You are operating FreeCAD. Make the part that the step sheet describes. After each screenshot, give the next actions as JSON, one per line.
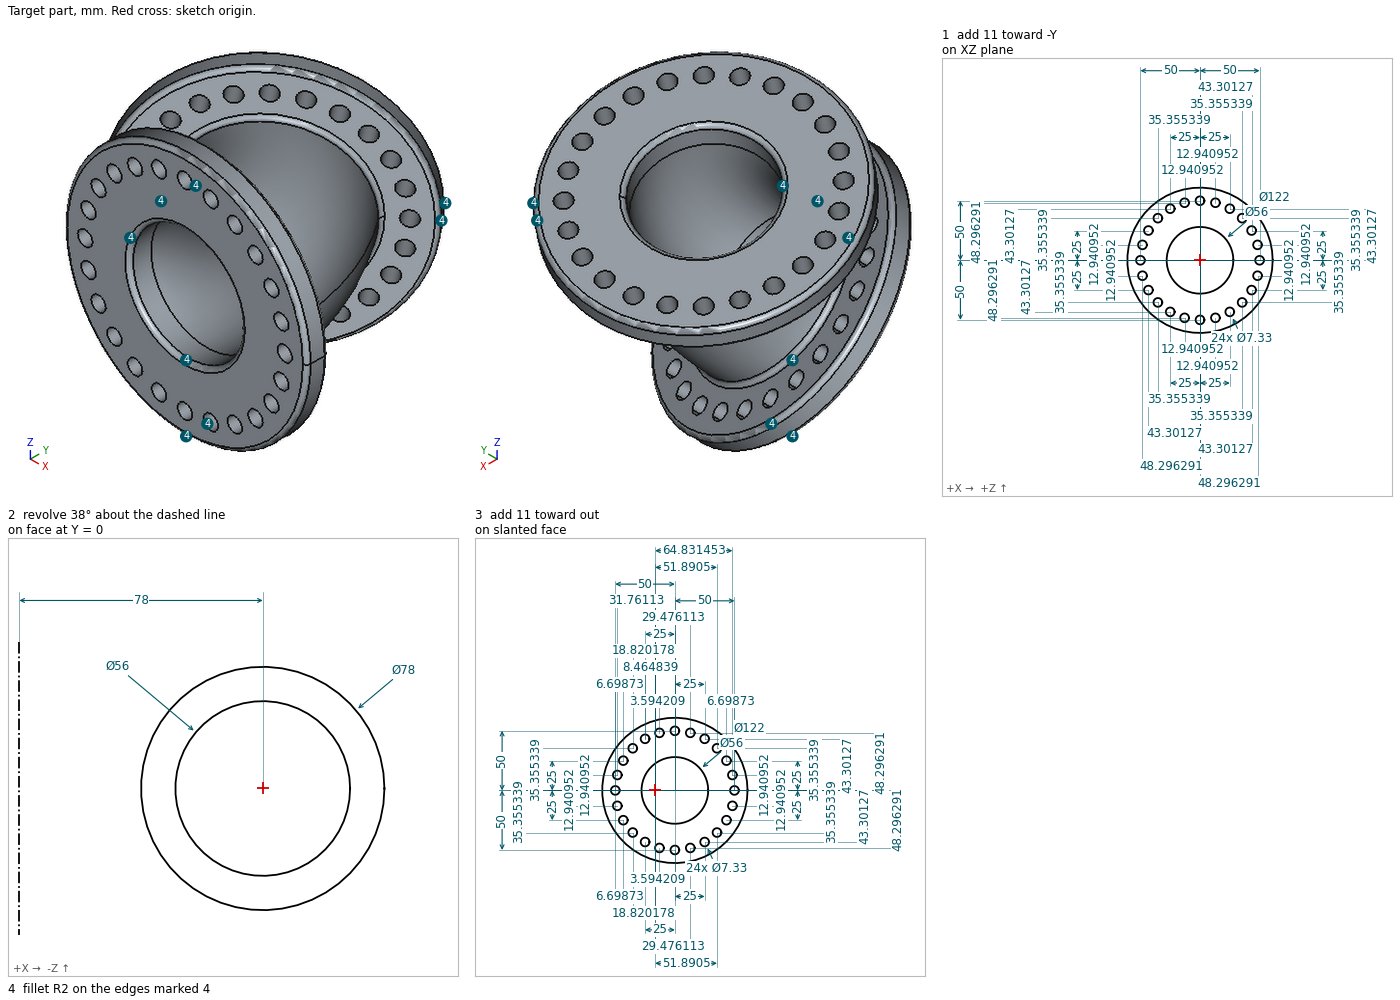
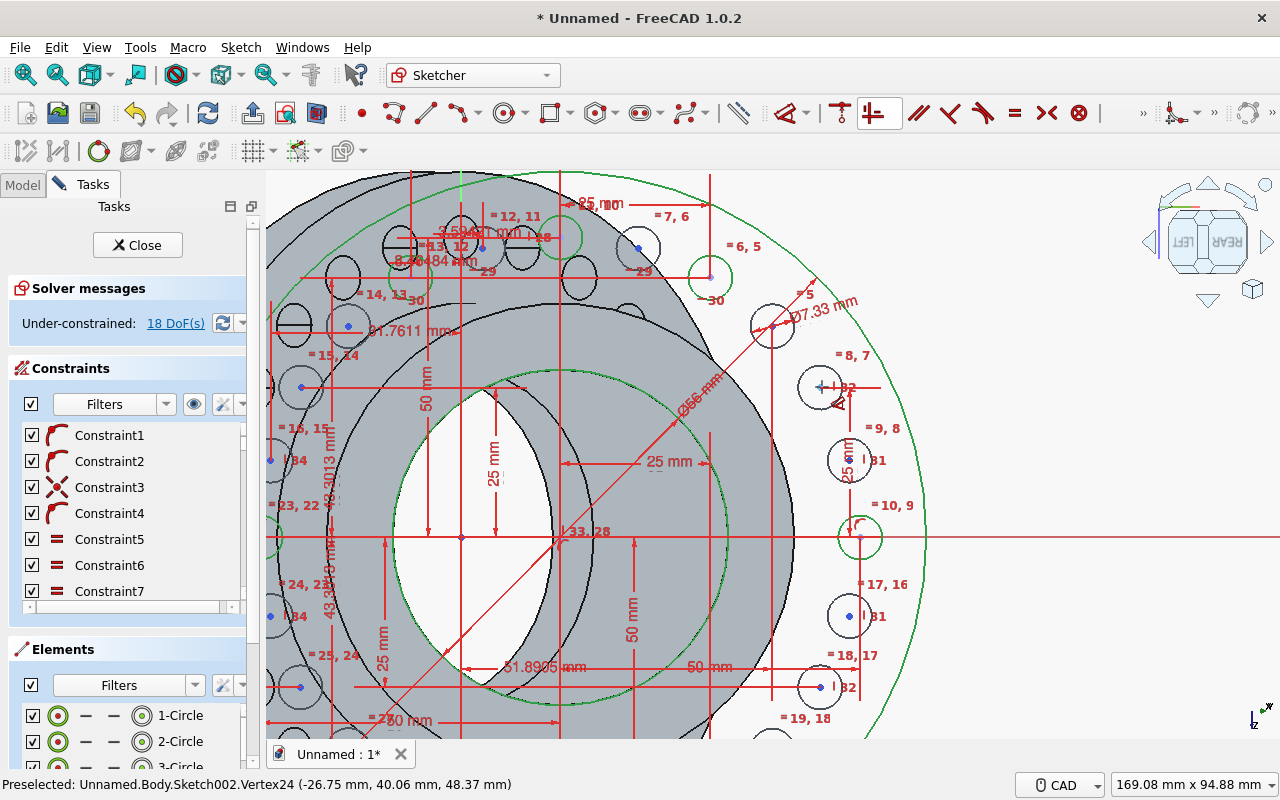
{"action": "left_click", "coordinate": [820, 388]}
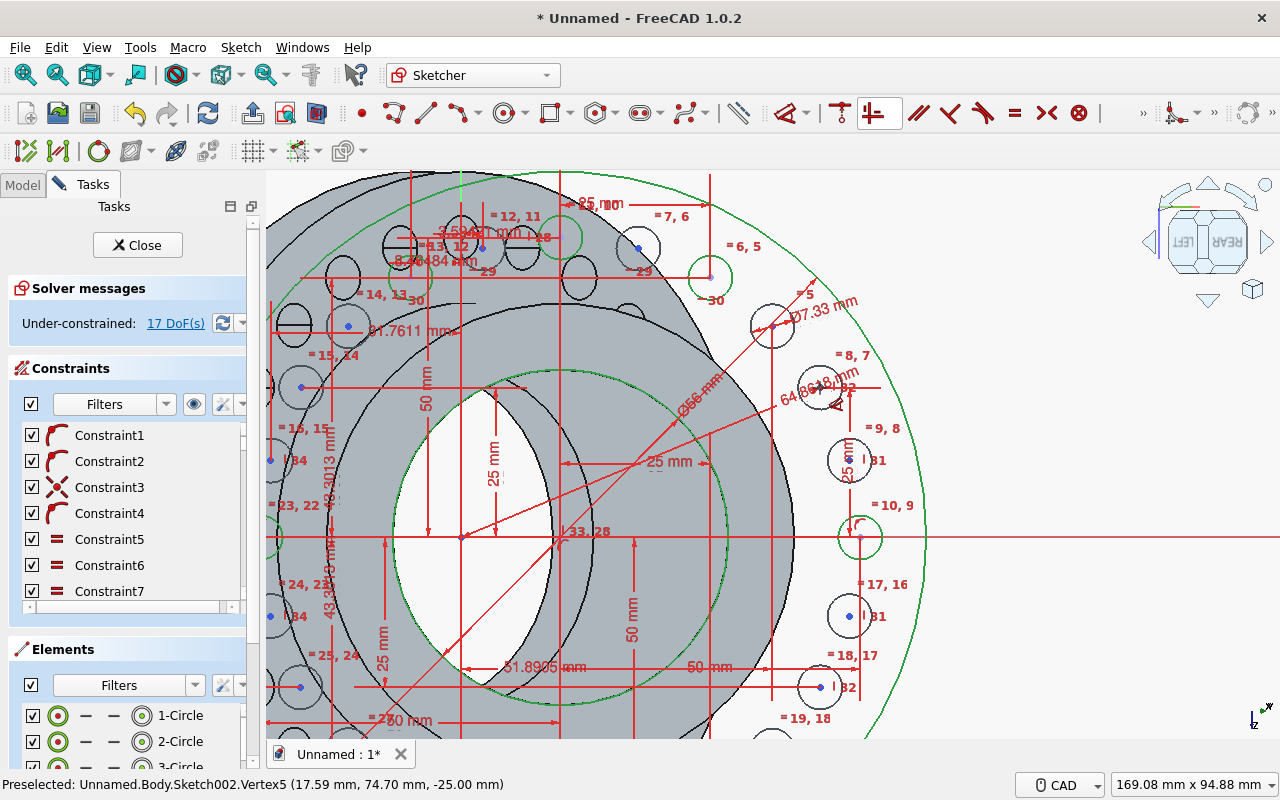
{"action": "left_click", "coordinate": [860, 537]}
{"action": "left_click", "coordinate": [840, 354]}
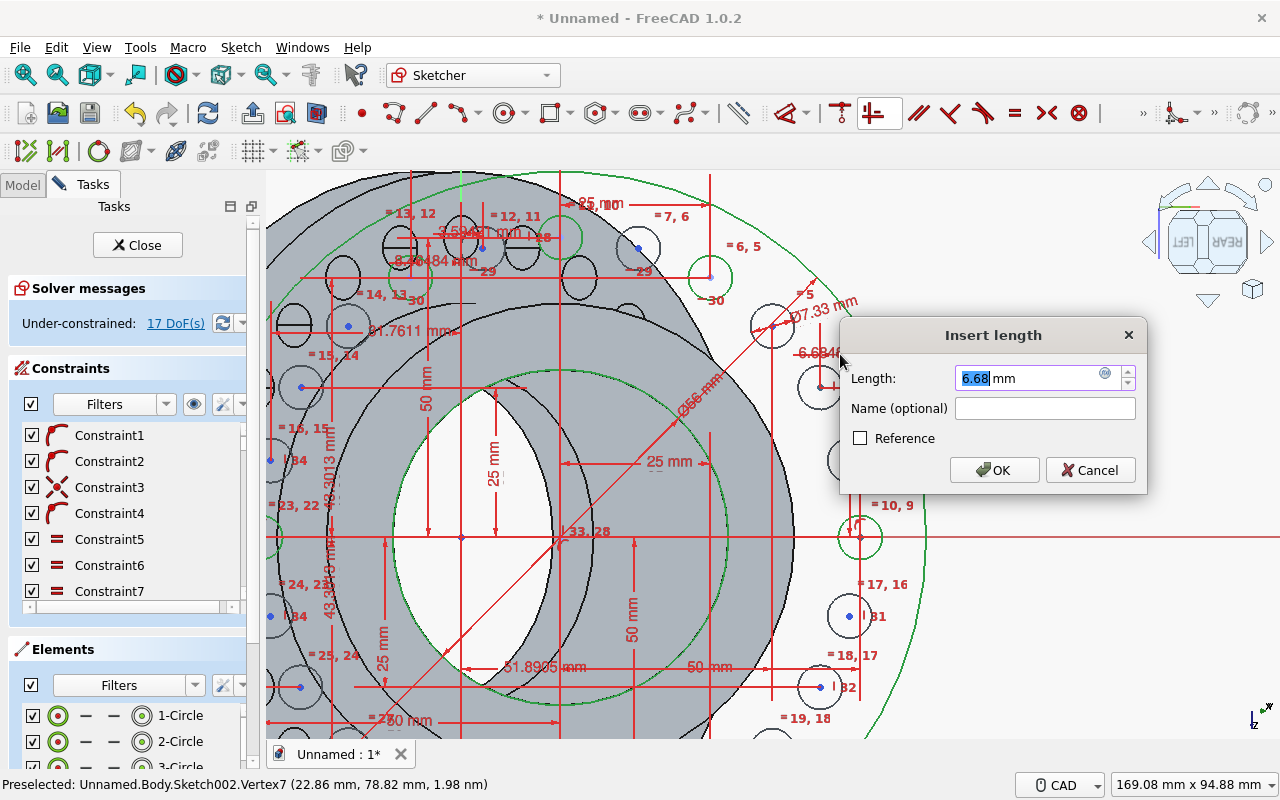
{"action": "type", "text": "6.69873"}
{"action": "key", "text": "Return"}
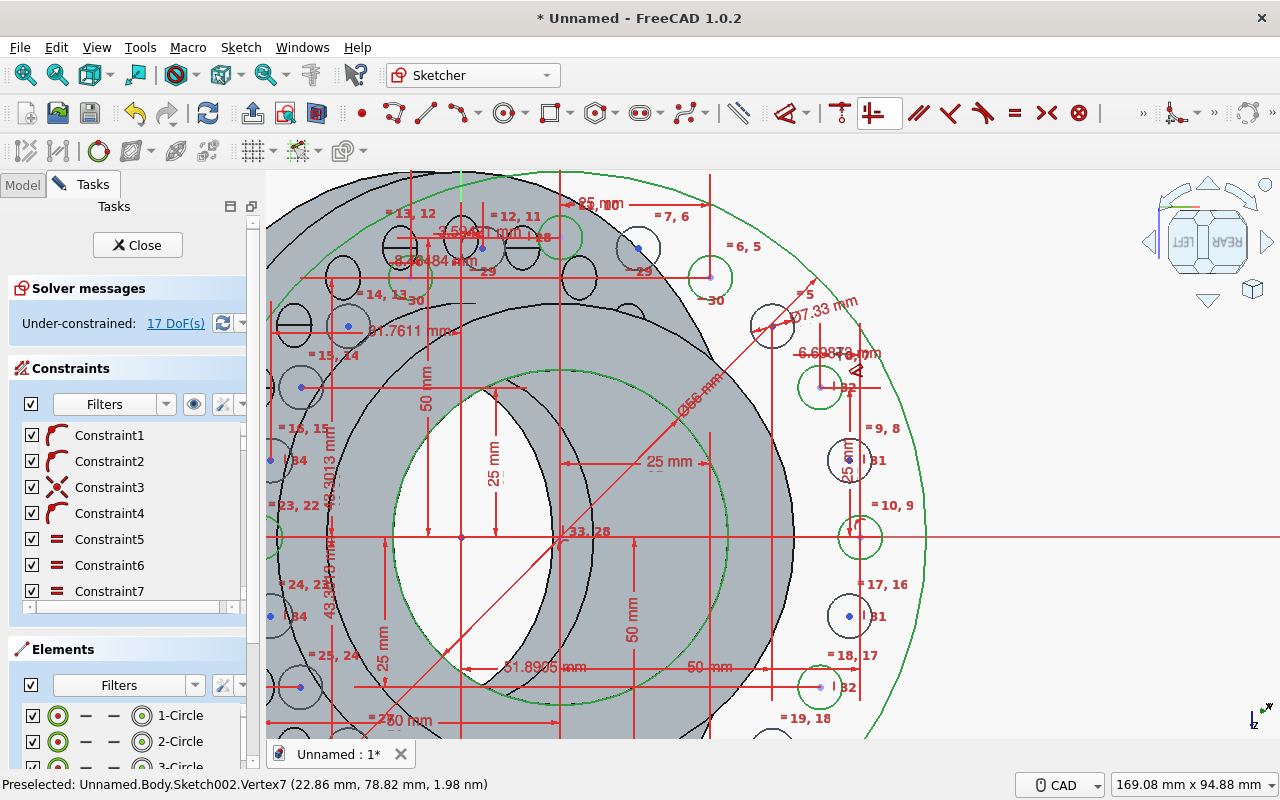
{"action": "left_click", "coordinate": [301, 388]}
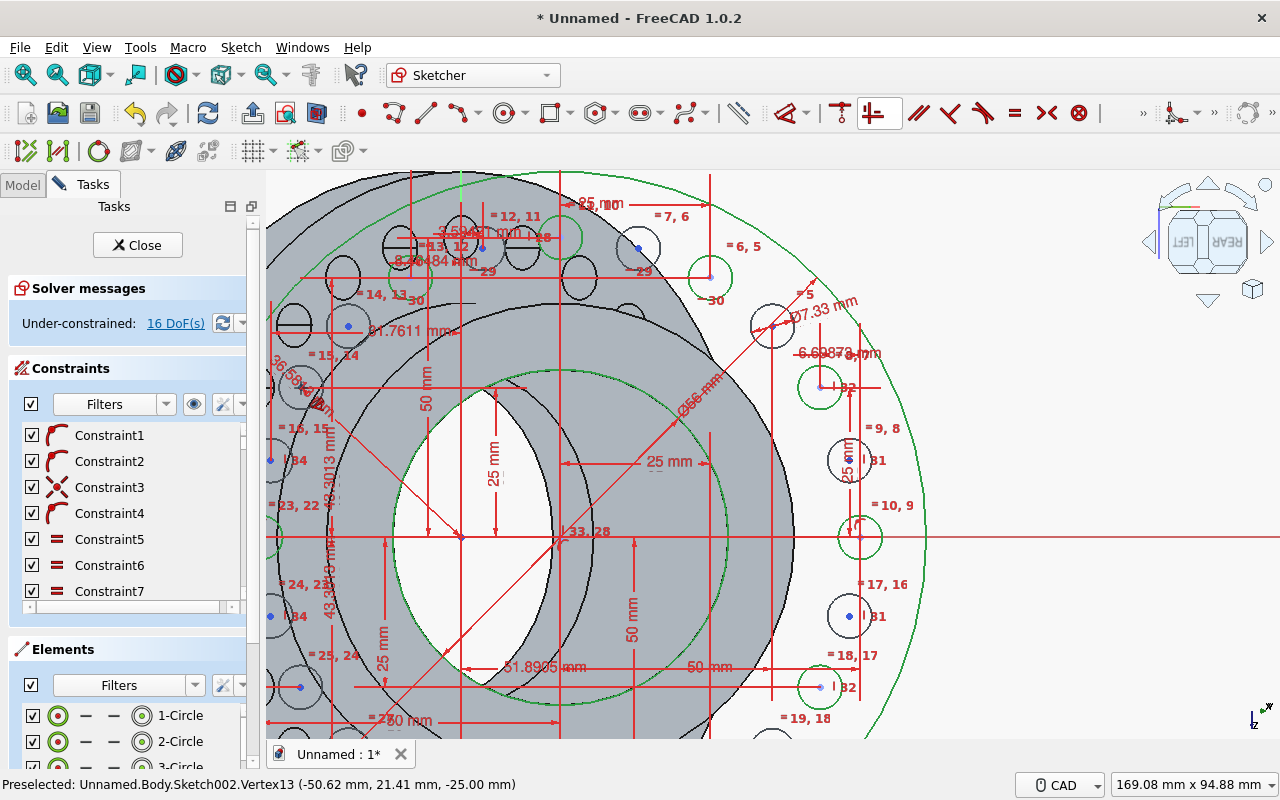
{"action": "scroll", "coordinate": [822, 387], "scroll_direction": "down", "scroll_amount": 4}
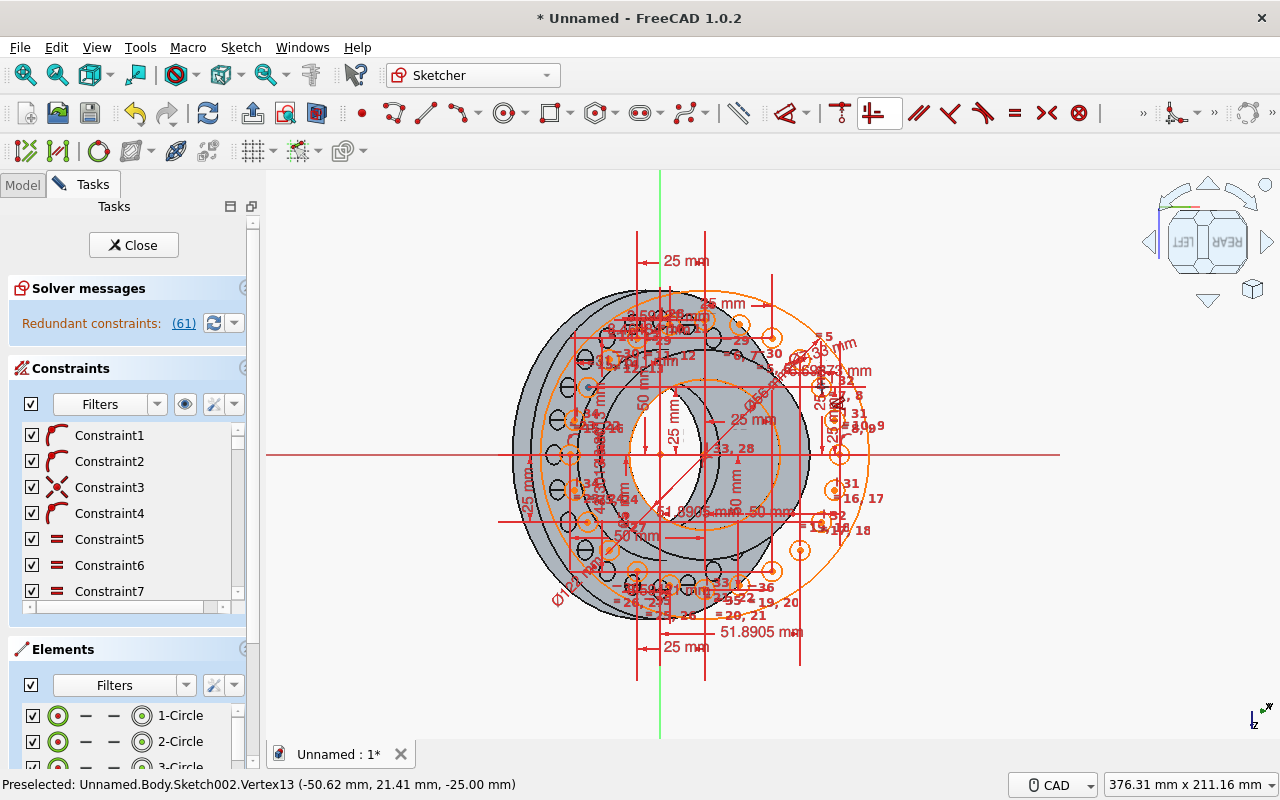
{"action": "scroll", "coordinate": [570, 455], "scroll_direction": "up", "scroll_amount": 4}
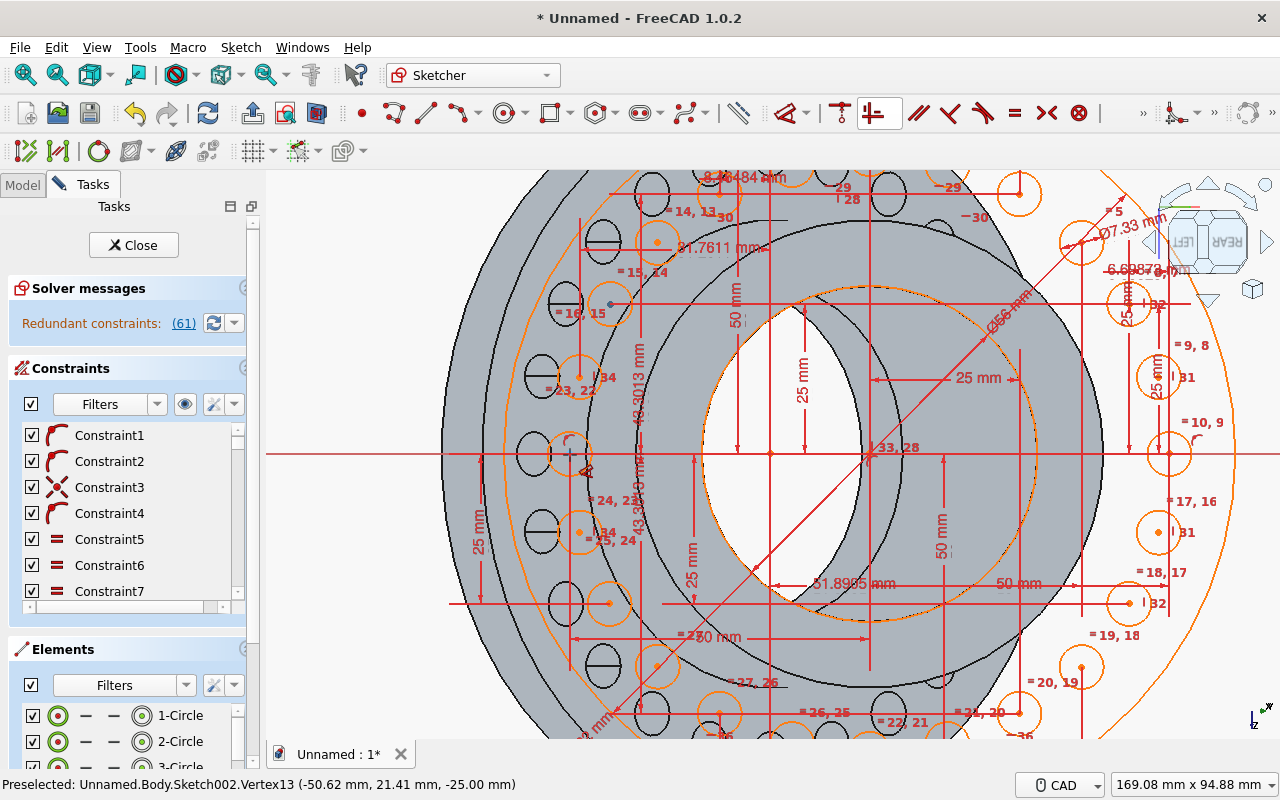
{"action": "left_click", "coordinate": [570, 454]}
{"action": "left_click", "coordinate": [590, 270]}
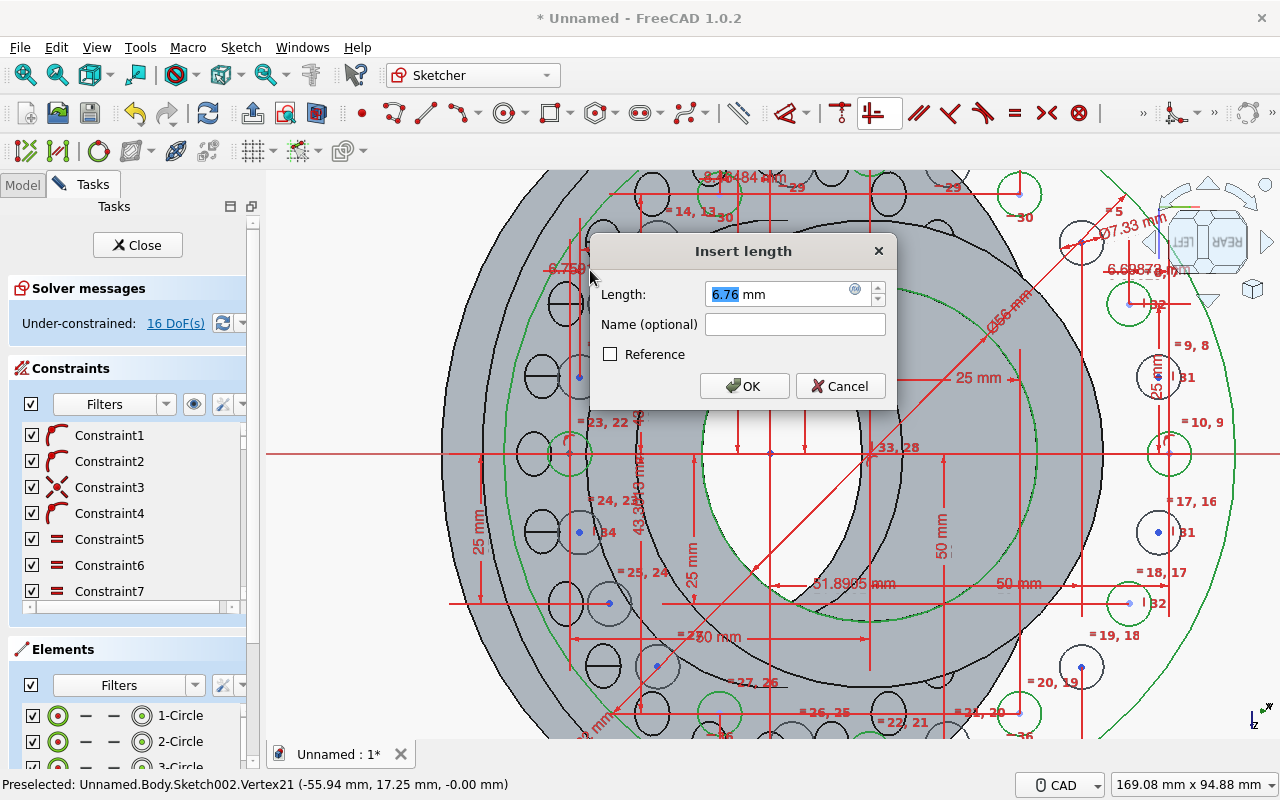
{"action": "type", "text": "6.69873"}
{"action": "key", "text": "Return"}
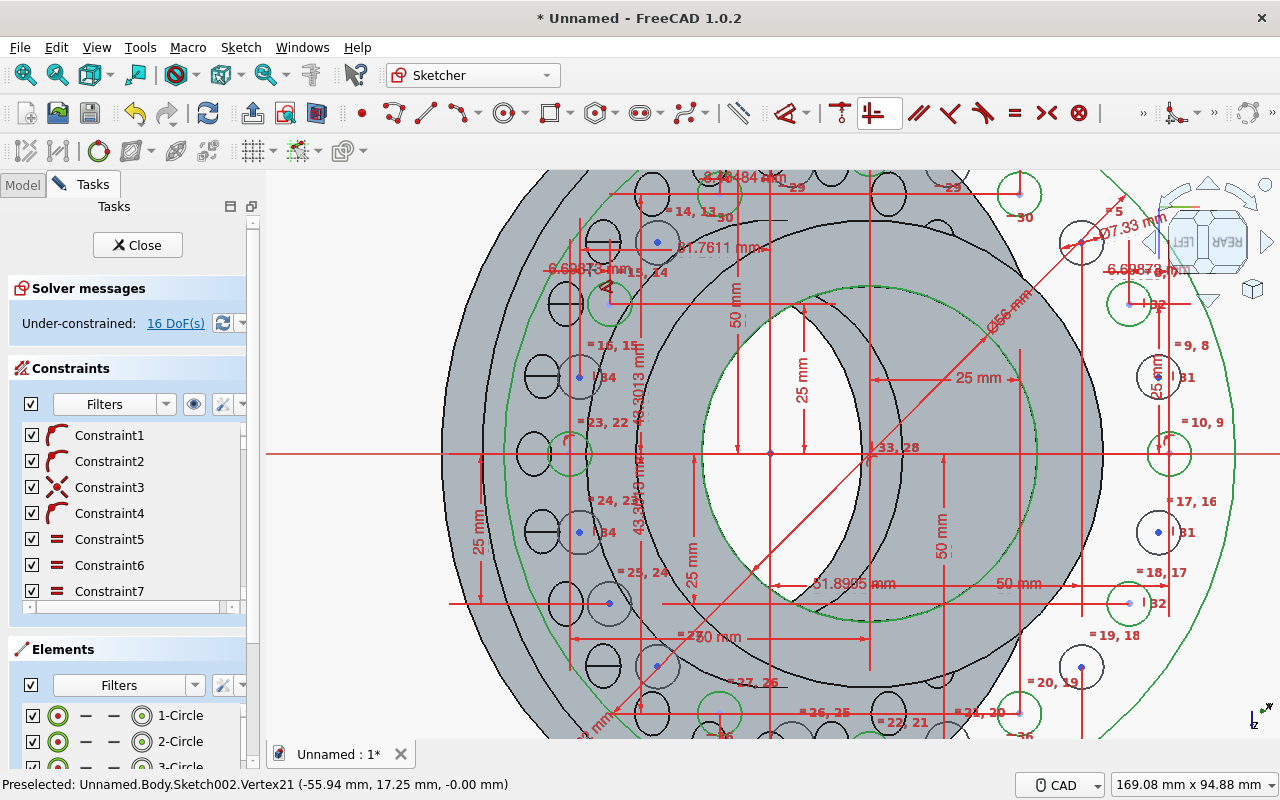
{"action": "left_click", "coordinate": [570, 454]}